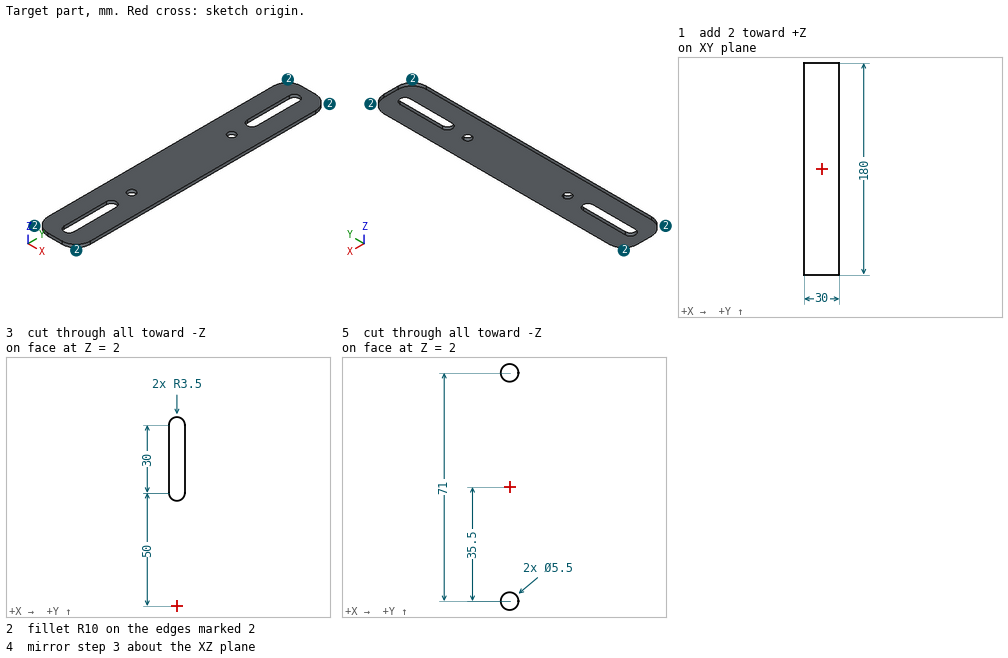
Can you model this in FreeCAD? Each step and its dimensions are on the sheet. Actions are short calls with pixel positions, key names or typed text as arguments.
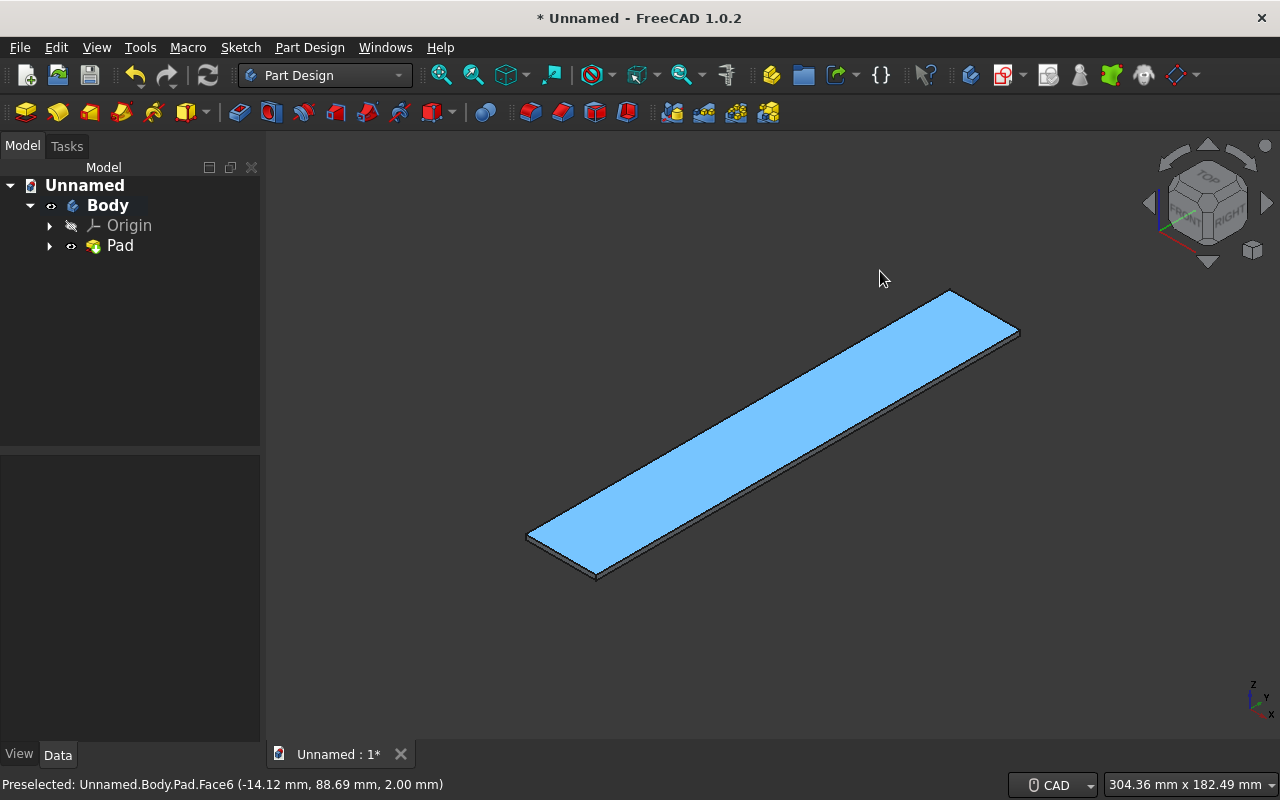
scroll(950, 291, up, 9)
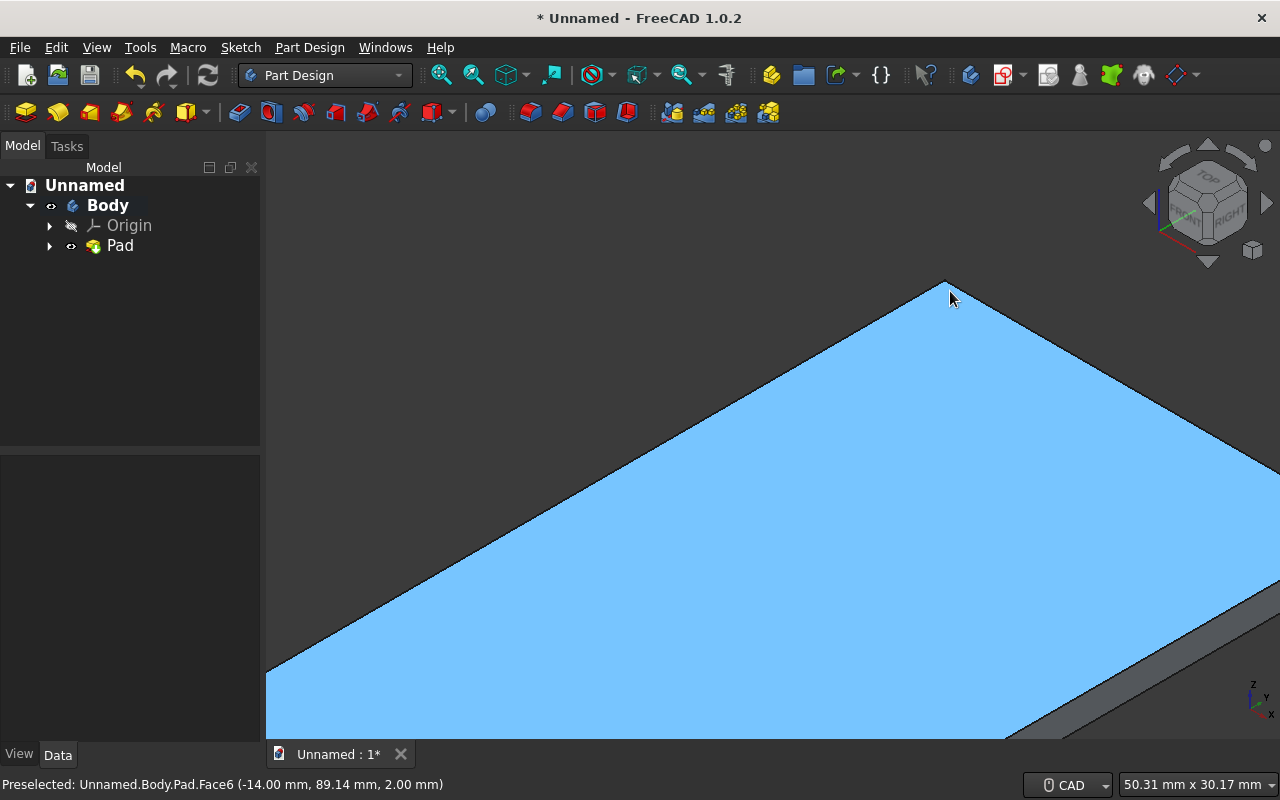
key(v)
key(f)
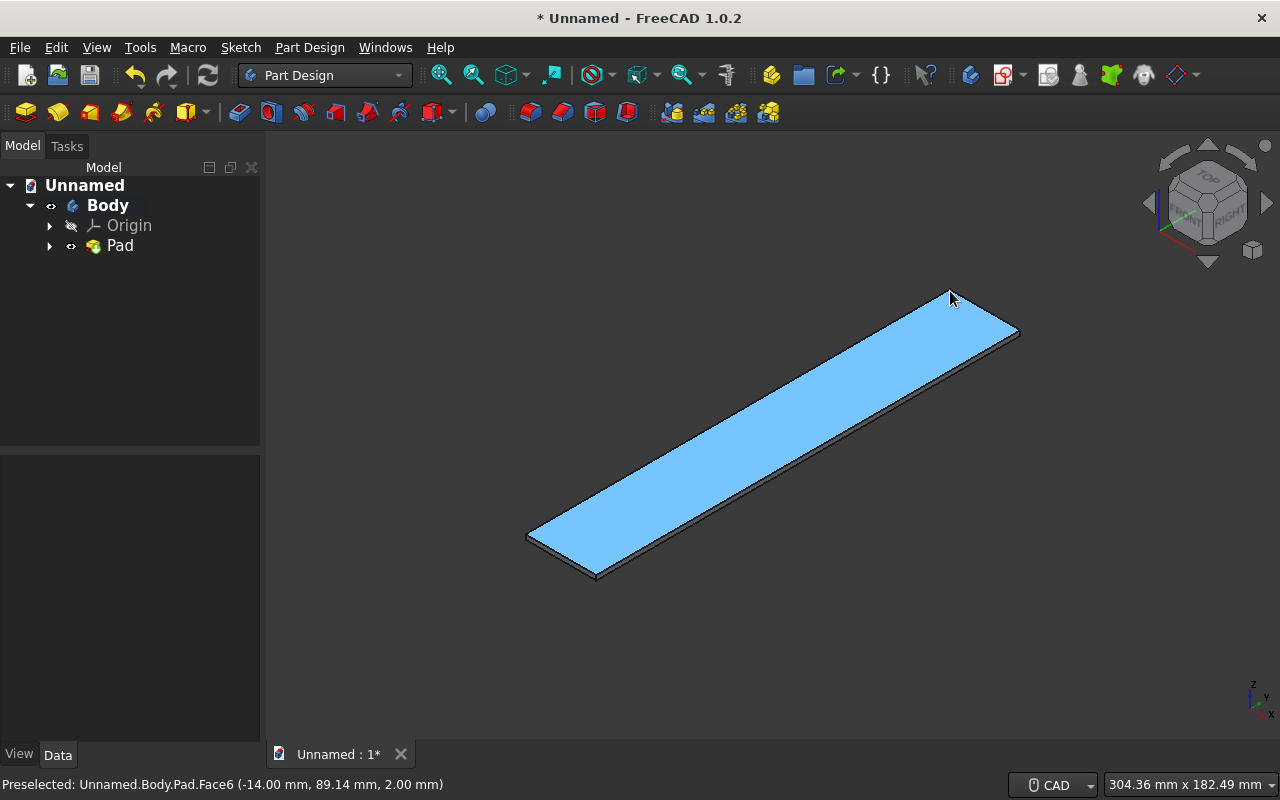
key(2)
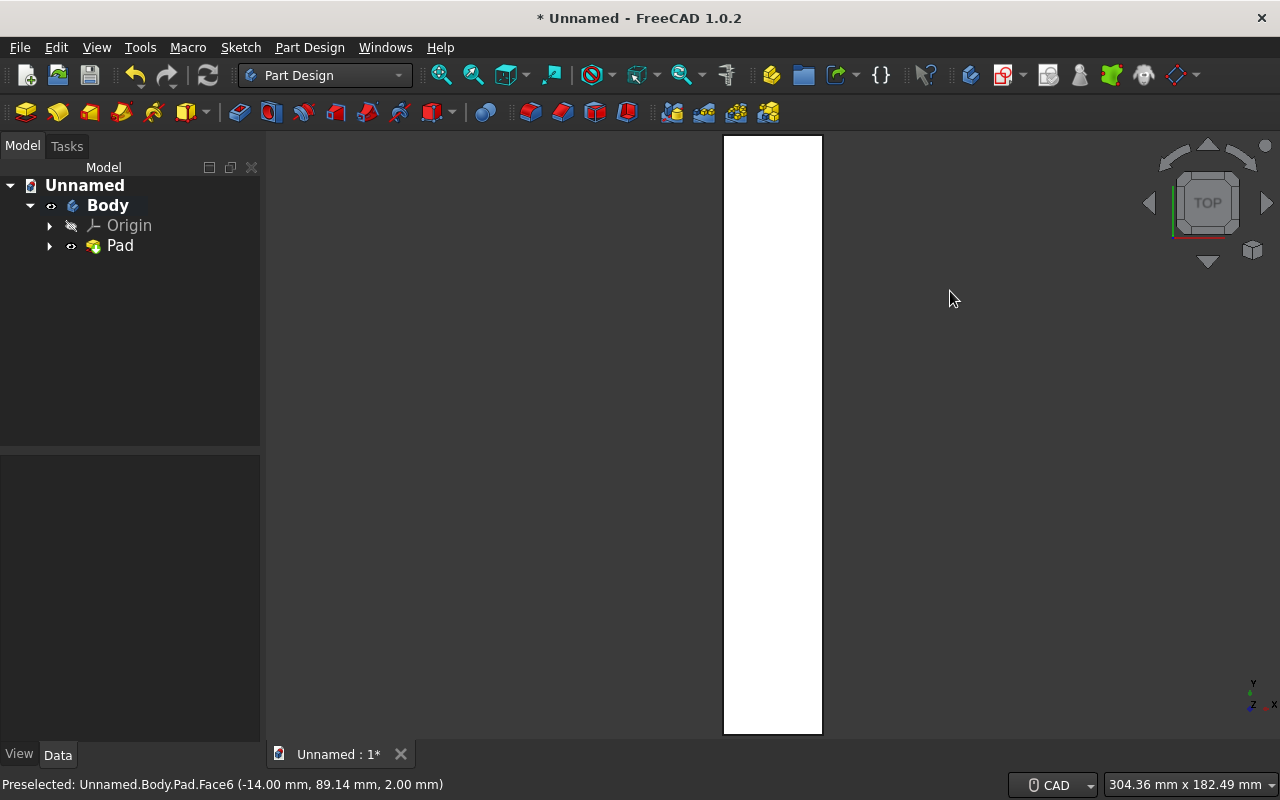
key(1)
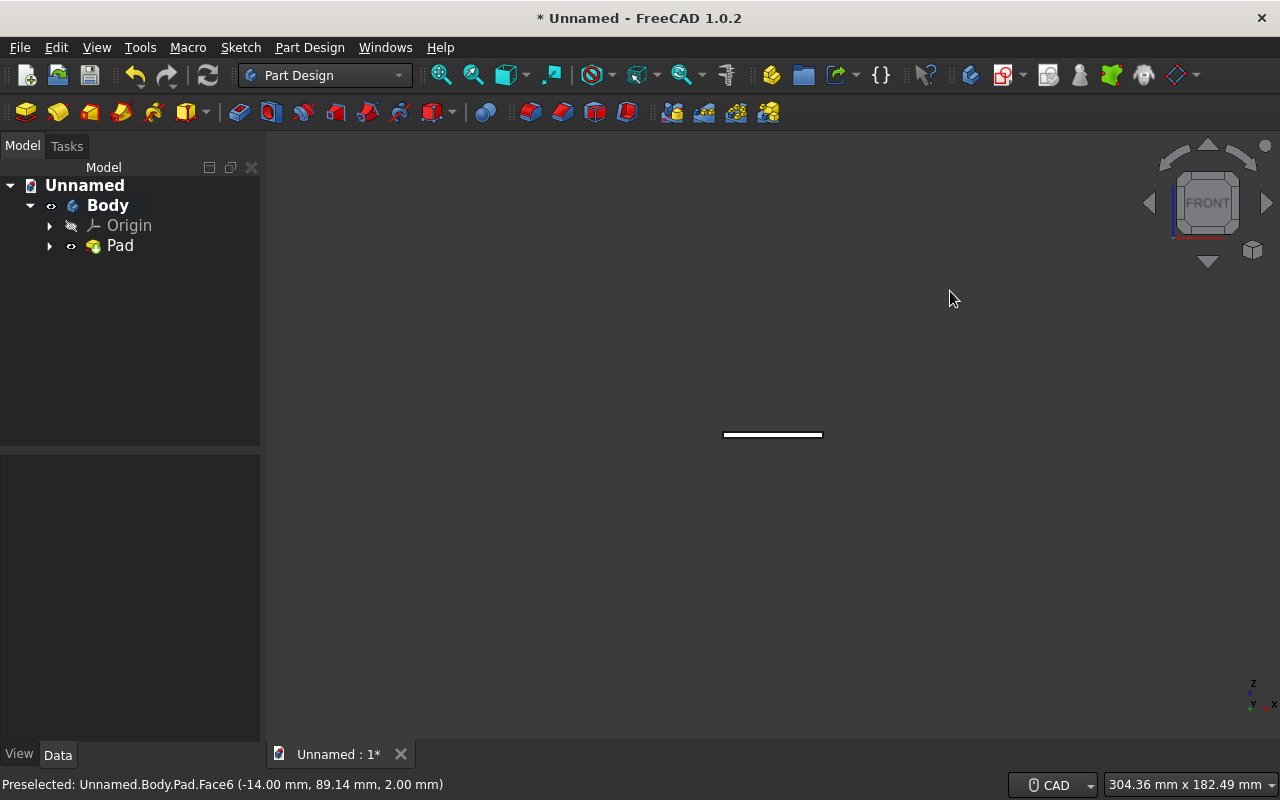
key(v)
key(f)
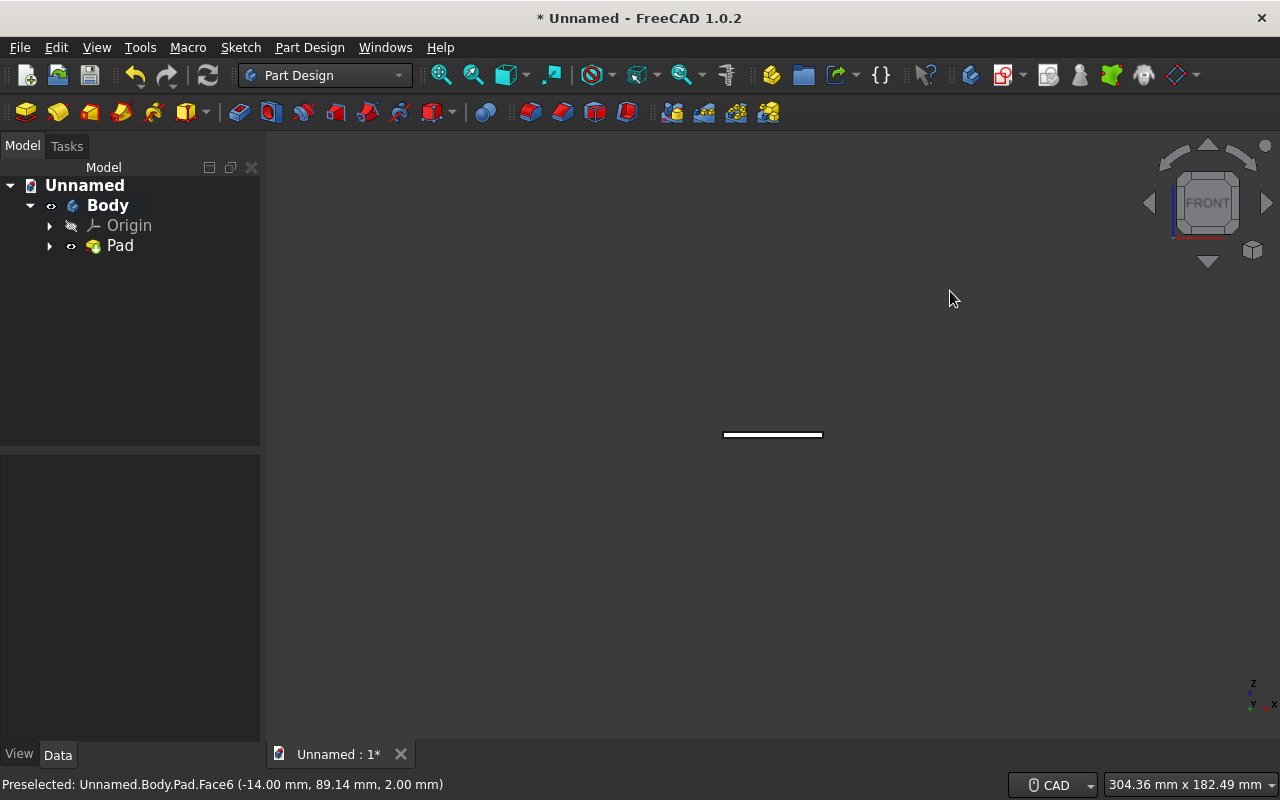
scroll(723, 434, up, 9)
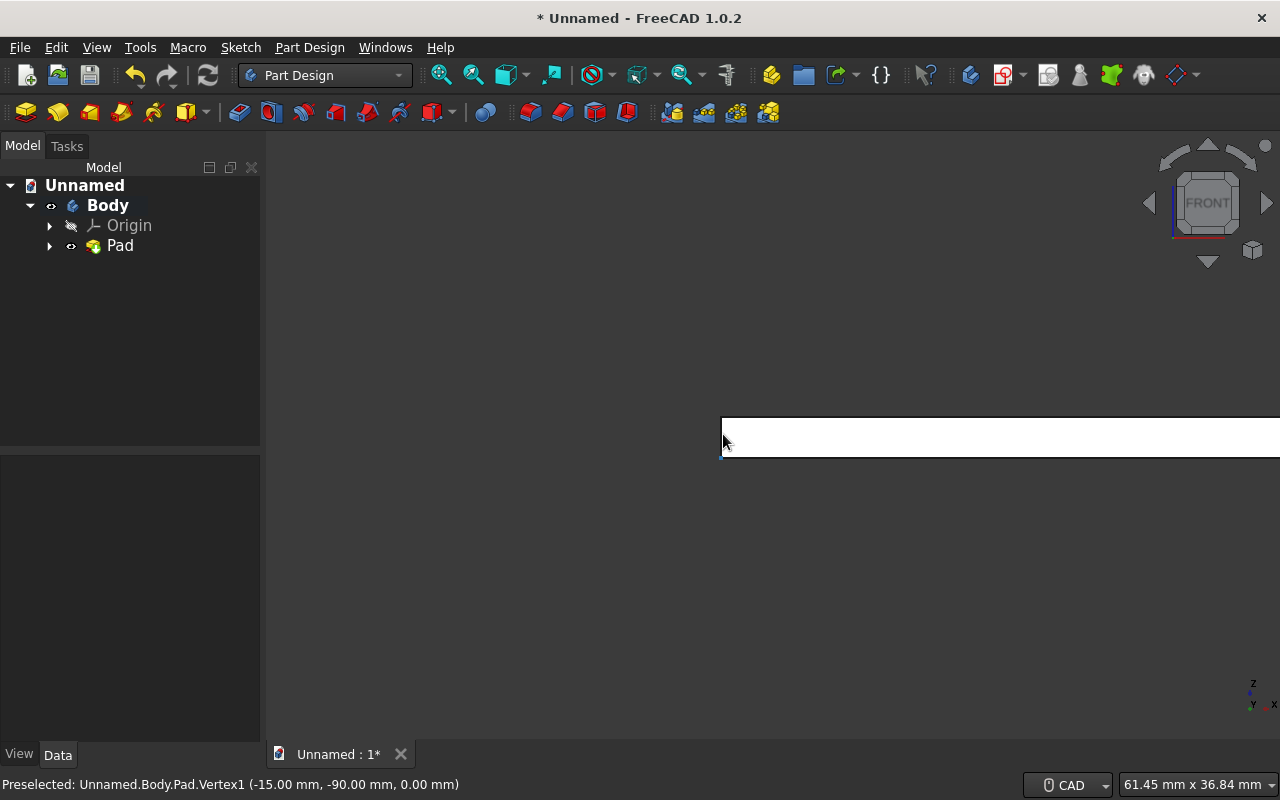
click(721, 437)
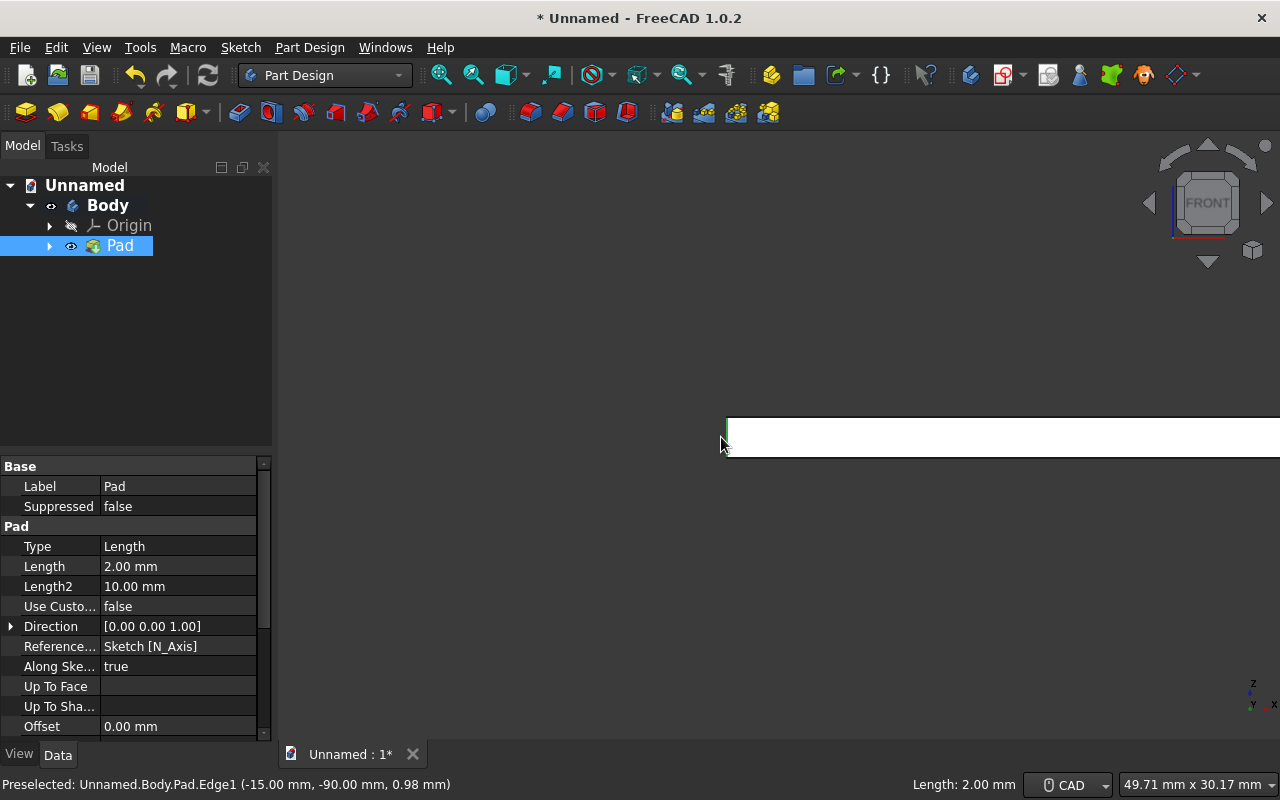
key(v)
key(f)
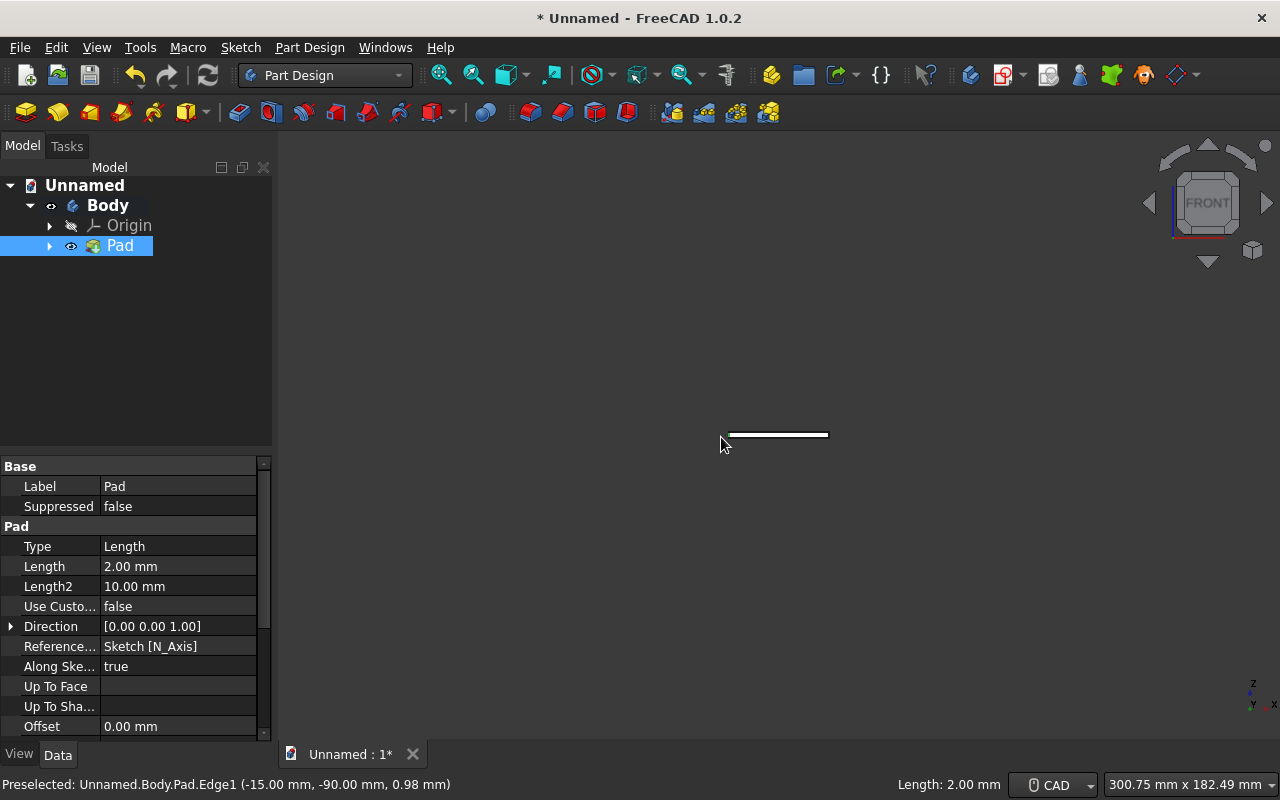
key(3)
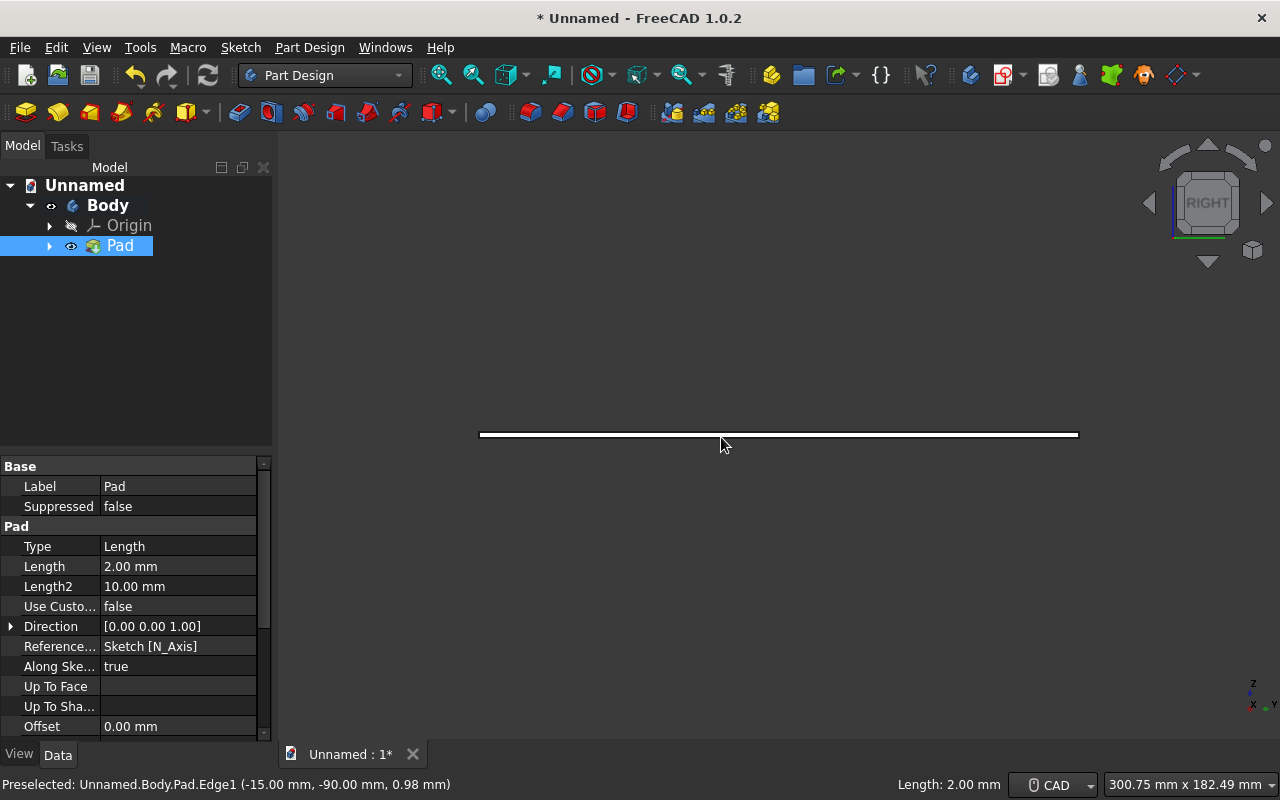
scroll(1079, 434, up, 9)